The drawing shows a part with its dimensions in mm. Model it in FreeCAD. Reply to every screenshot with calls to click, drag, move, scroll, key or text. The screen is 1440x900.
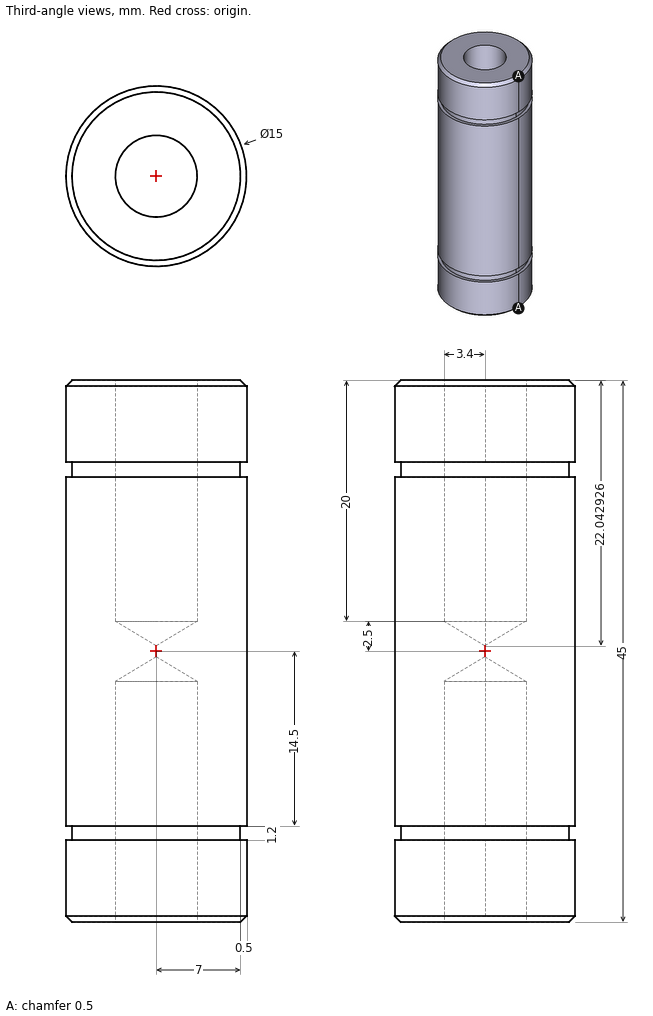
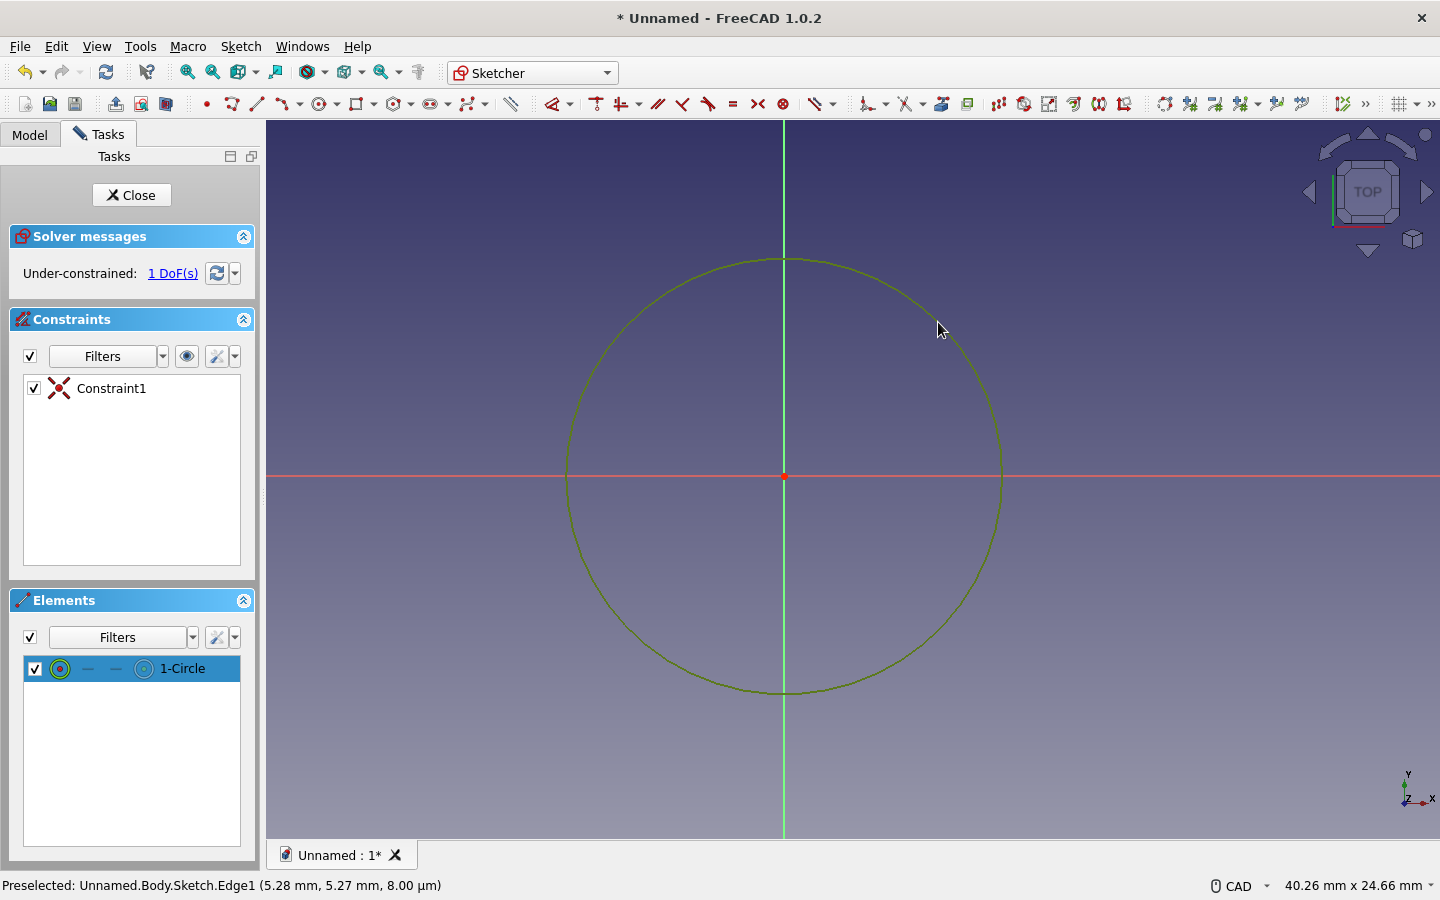
key(k)
key(o)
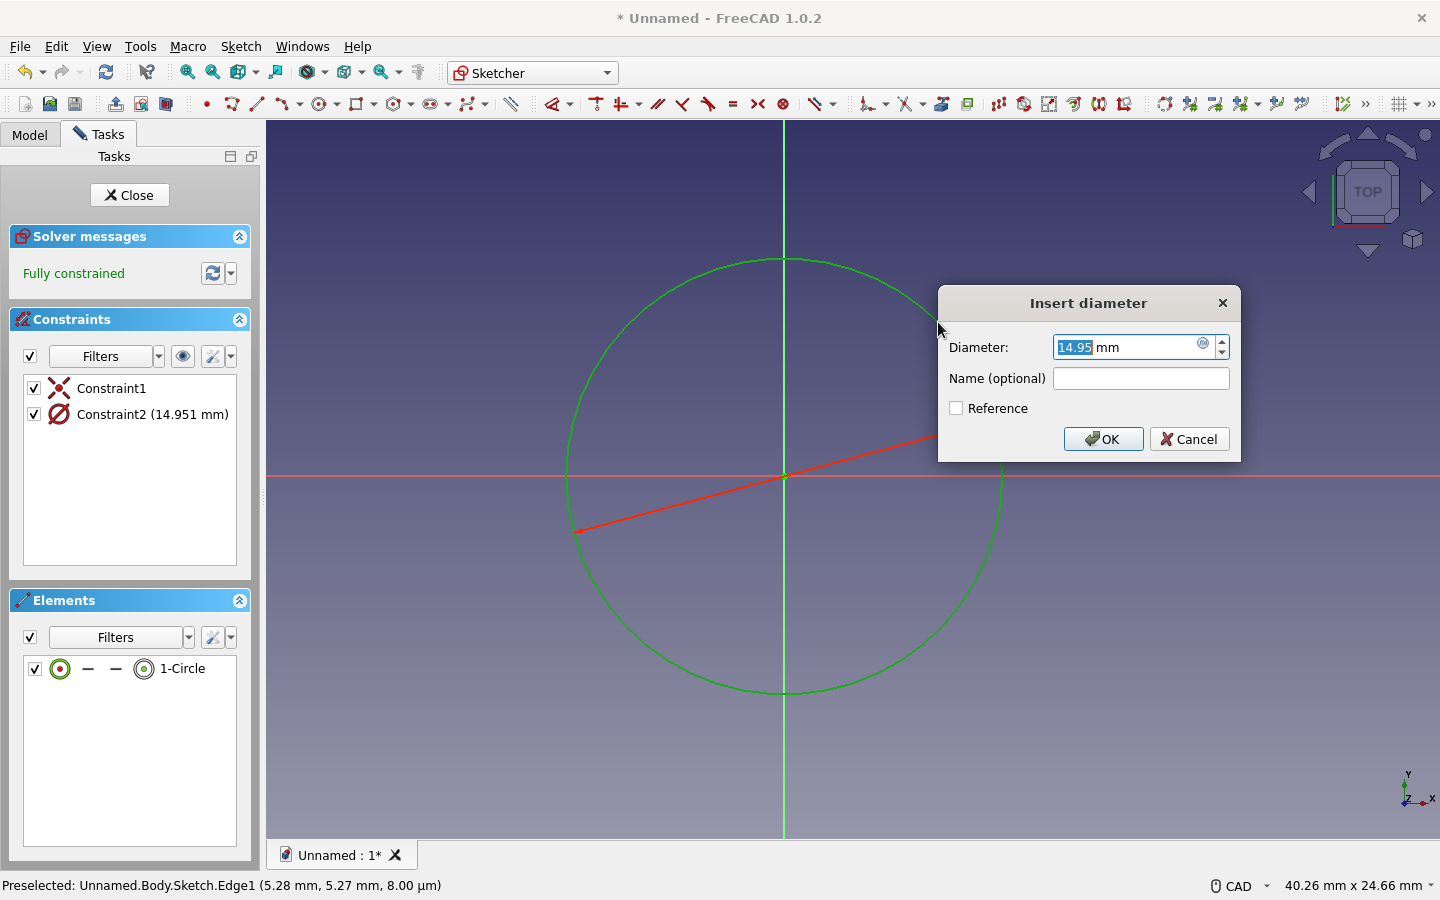
text(15)
key(Return)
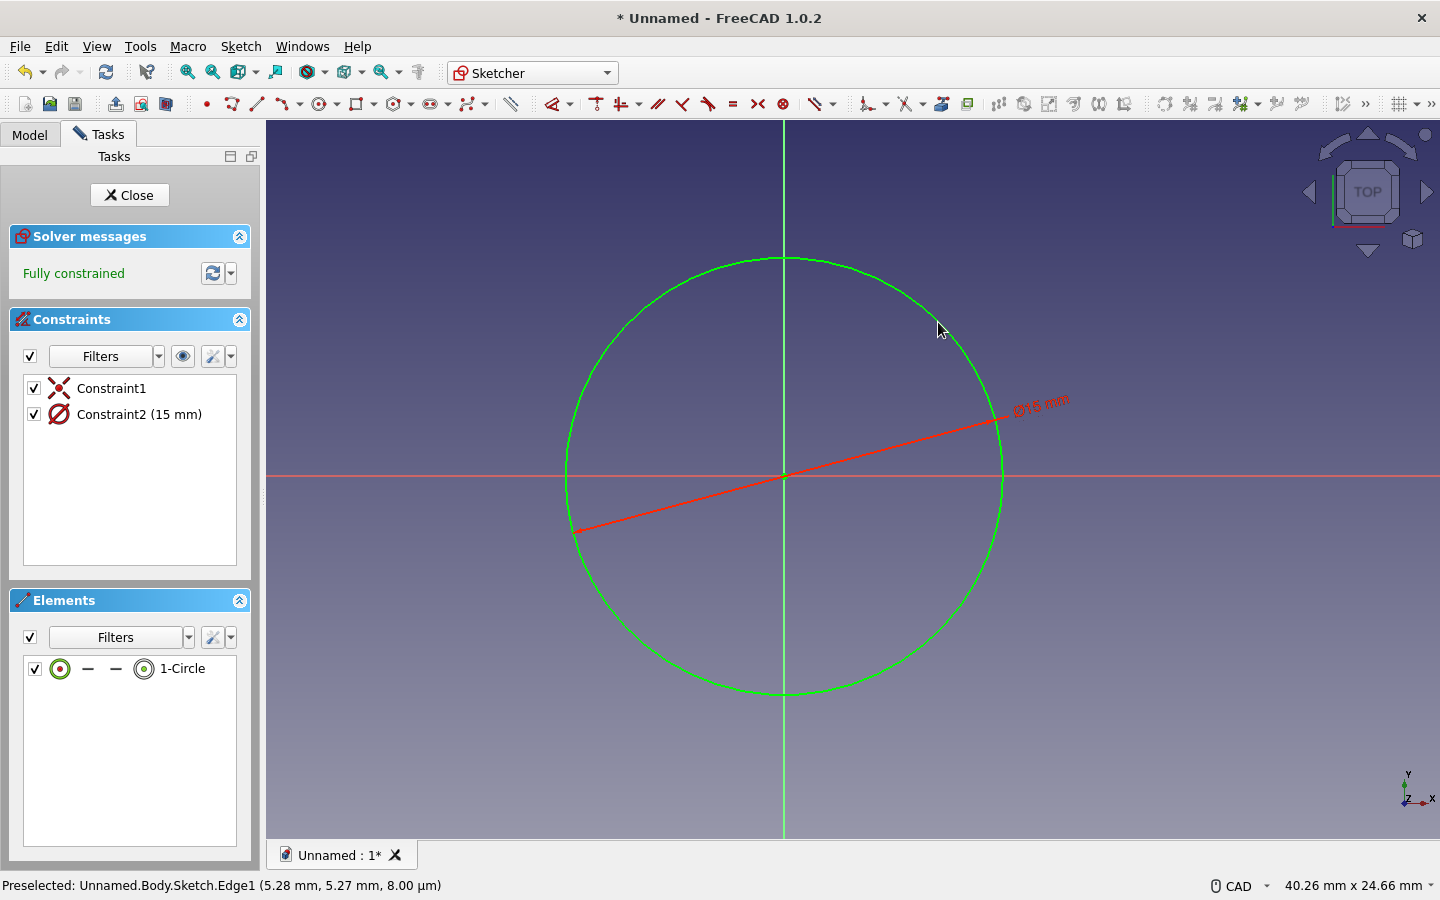
click(130, 195)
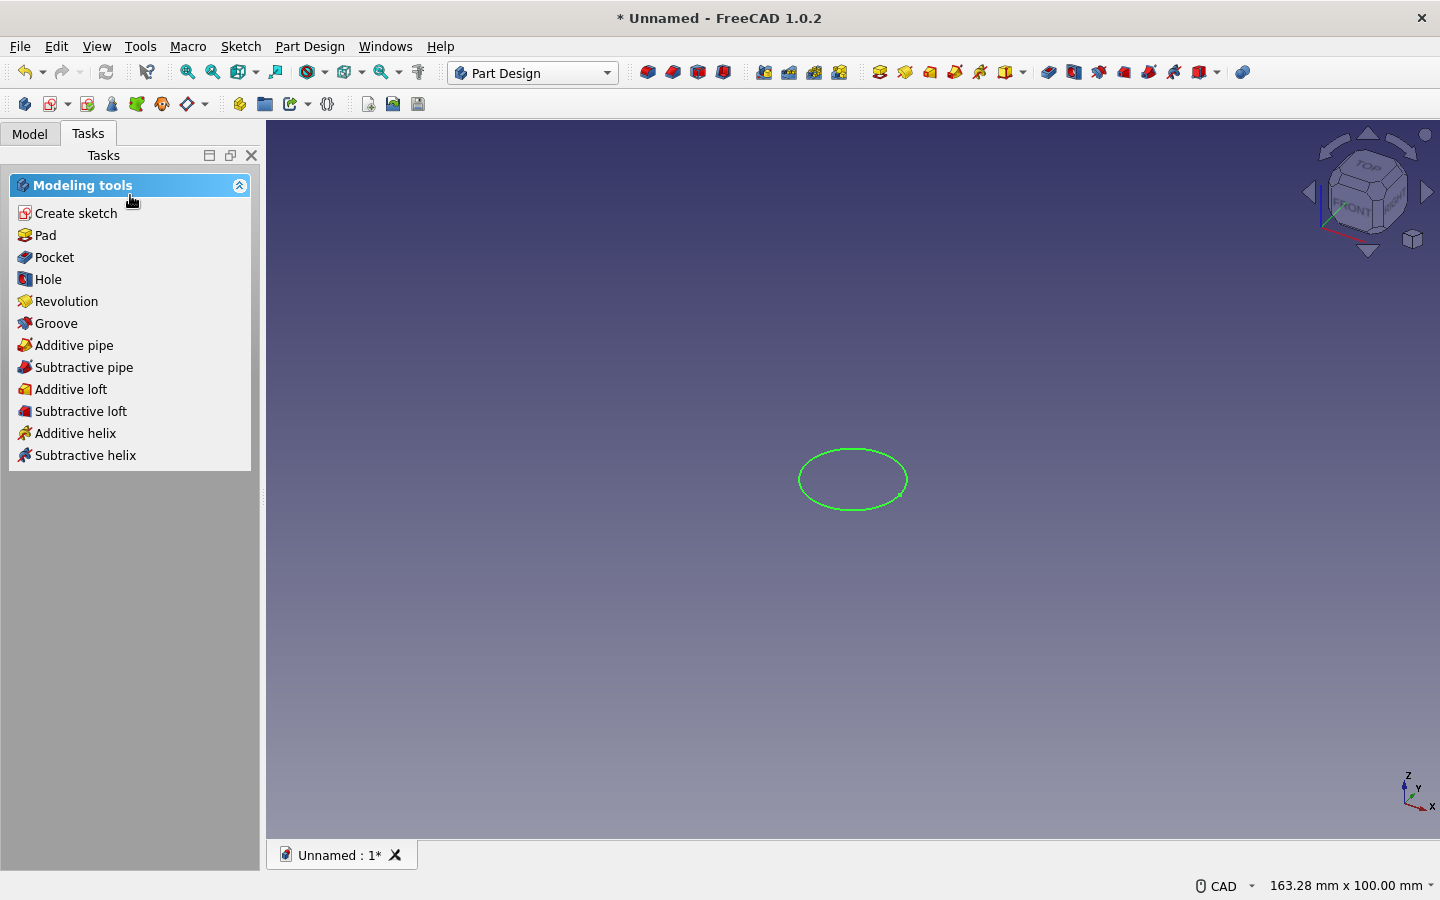
click(880, 72)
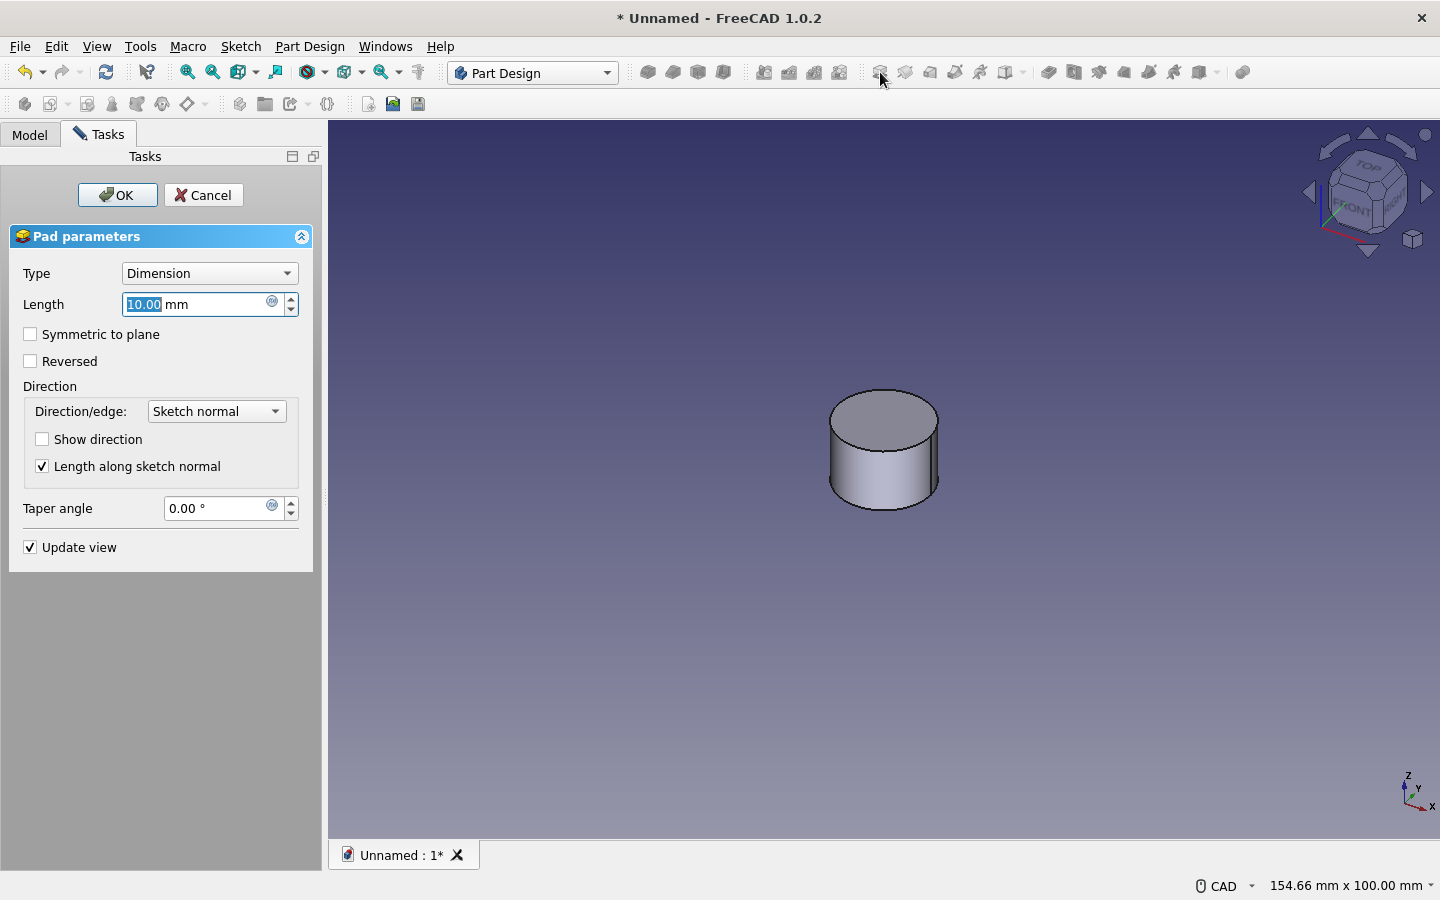
text(45)
key(Tab)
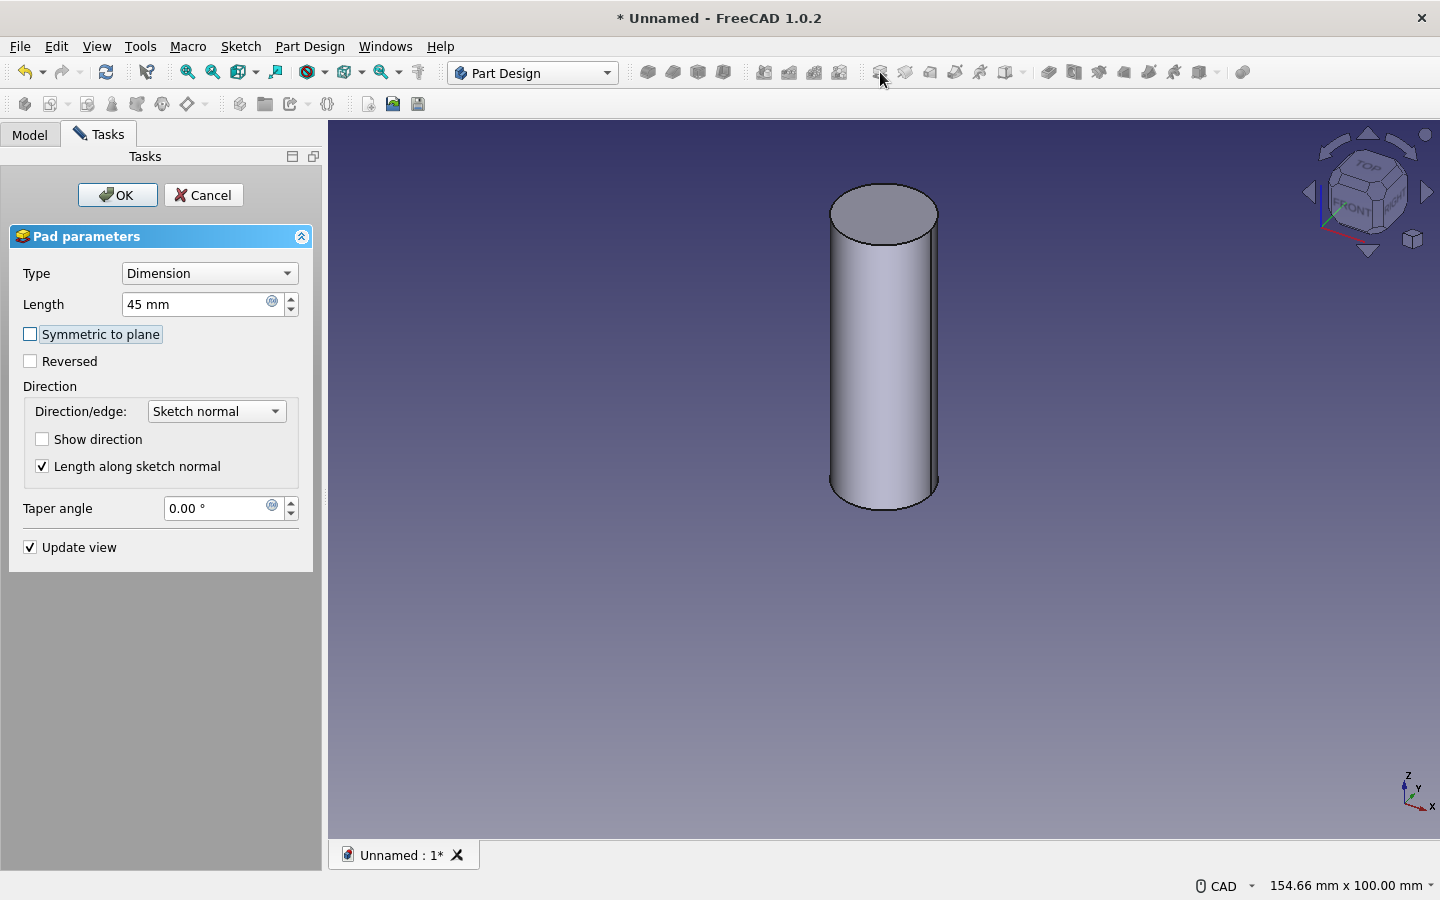
click(31, 334)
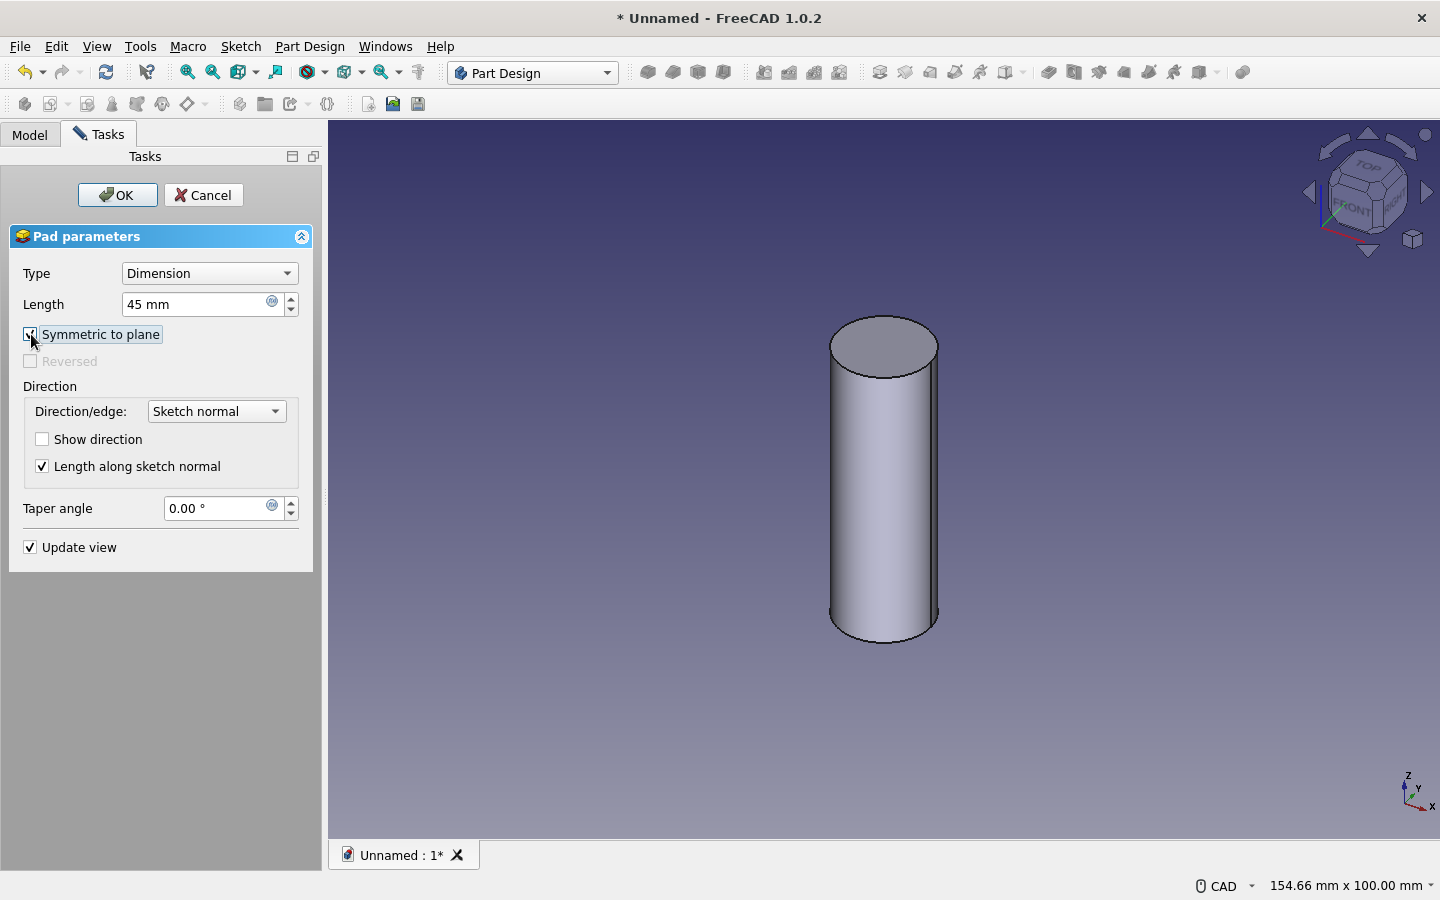
click(118, 195)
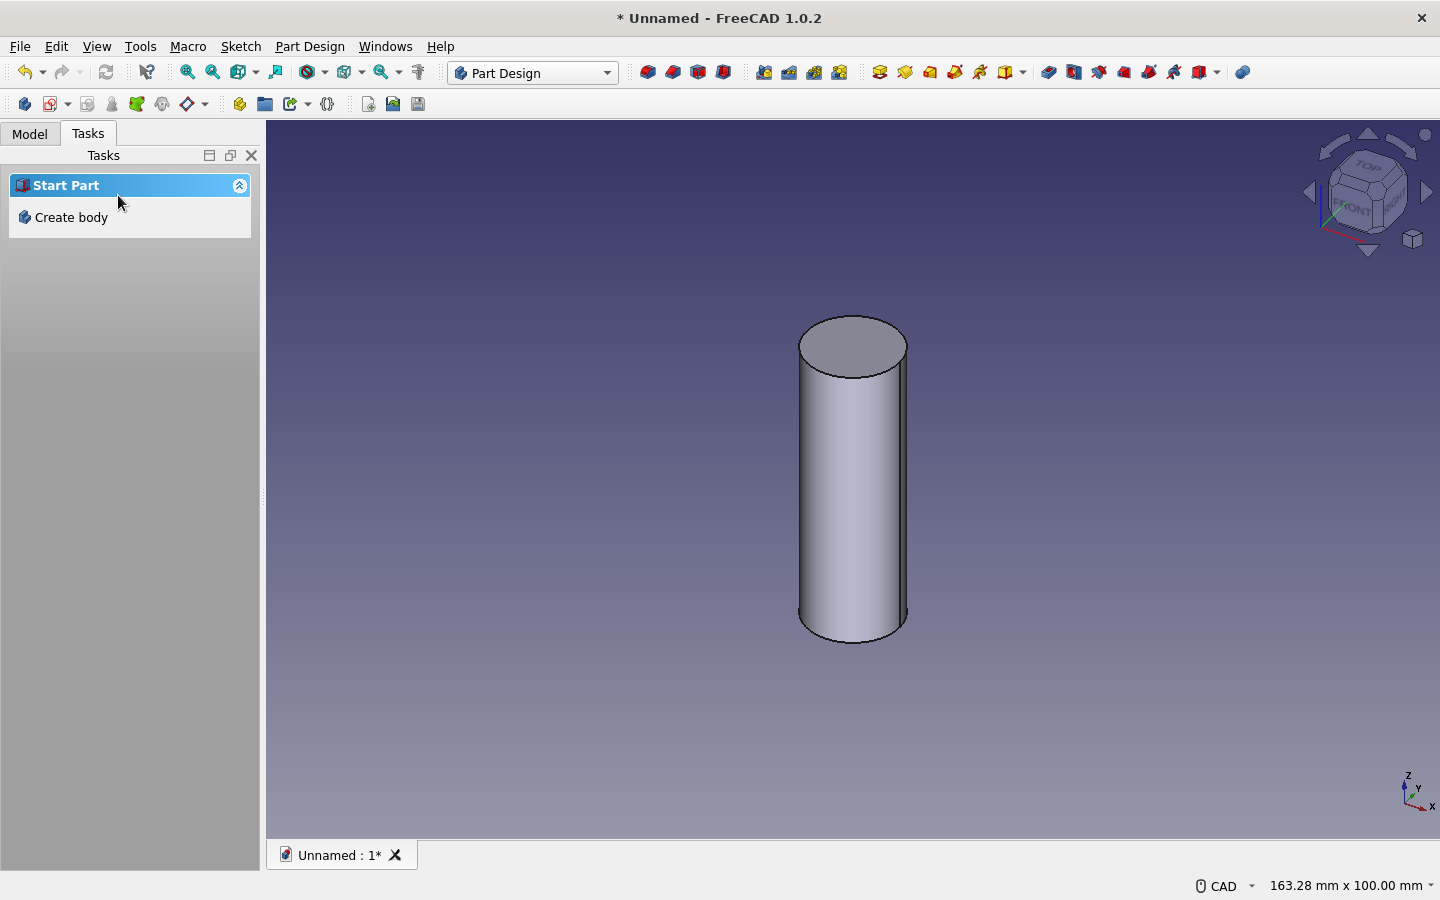
click(50, 104)